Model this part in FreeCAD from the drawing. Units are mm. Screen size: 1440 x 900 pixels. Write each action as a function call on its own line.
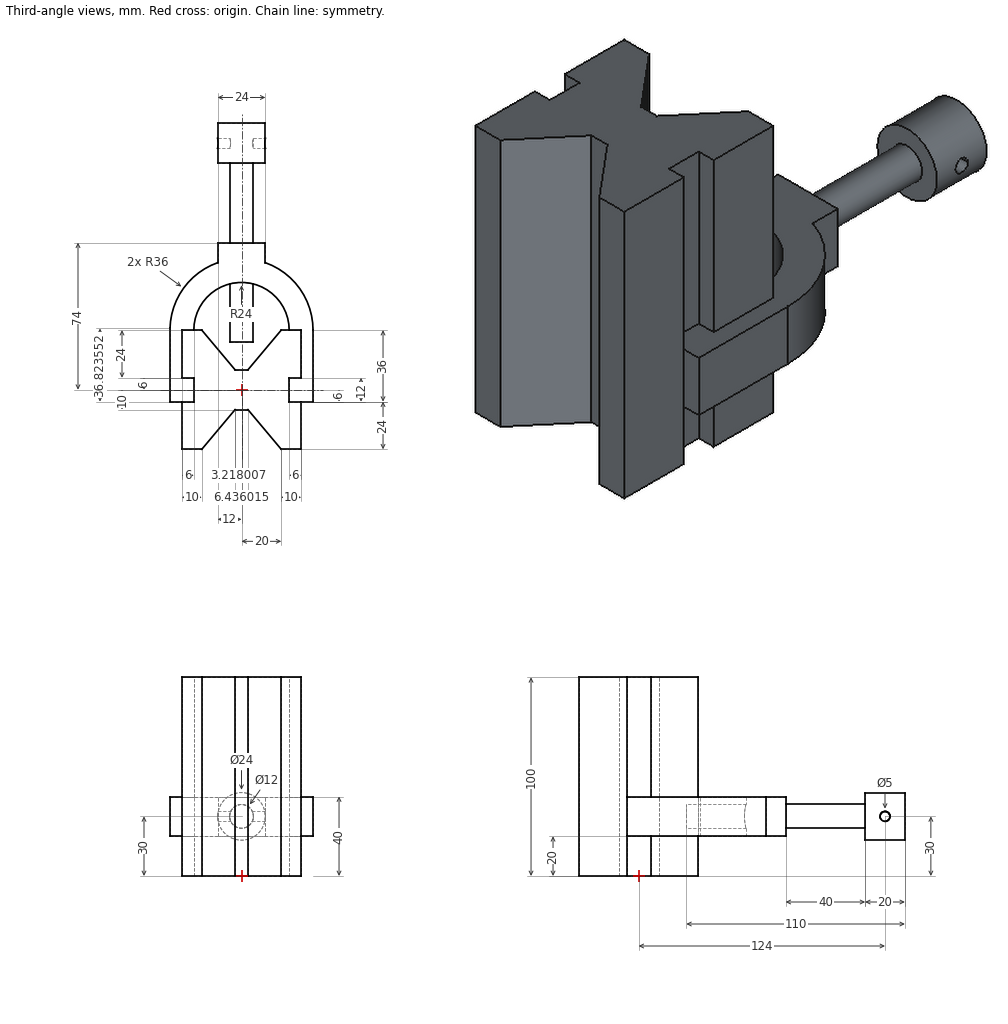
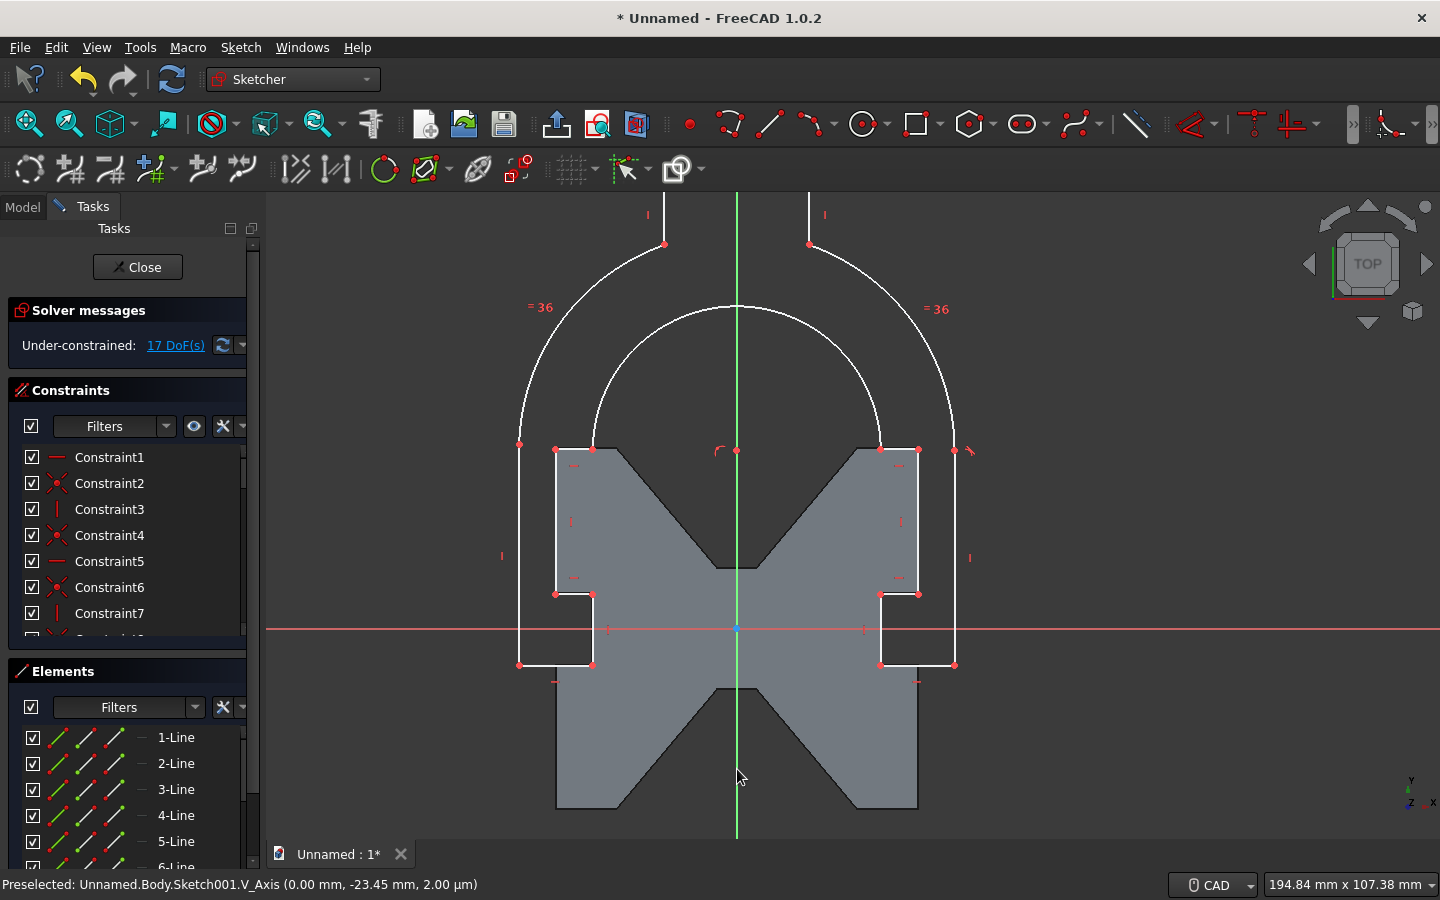
click(593, 666)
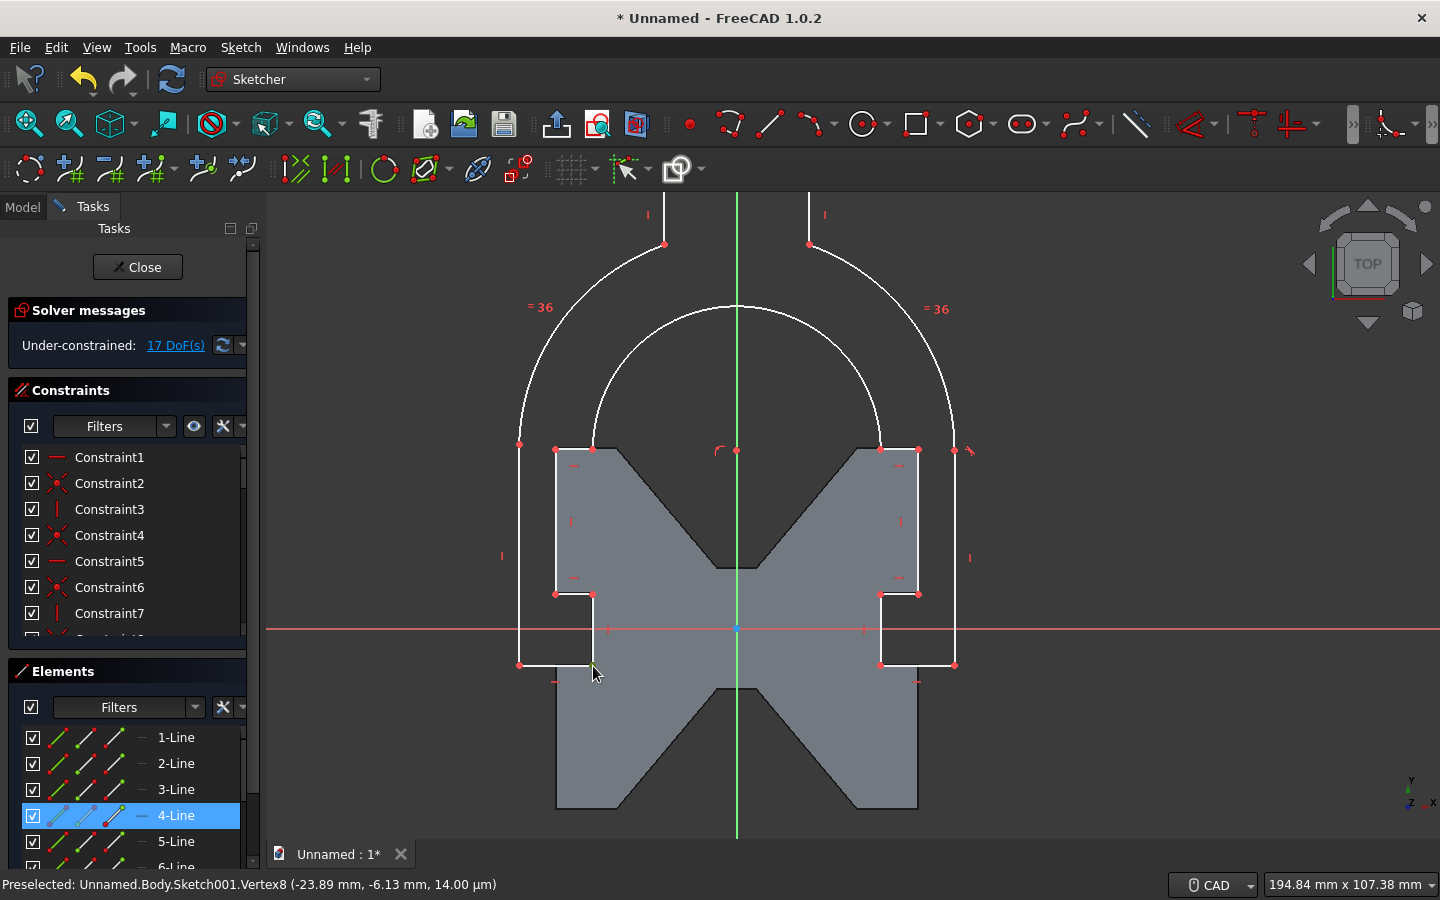
click(881, 666)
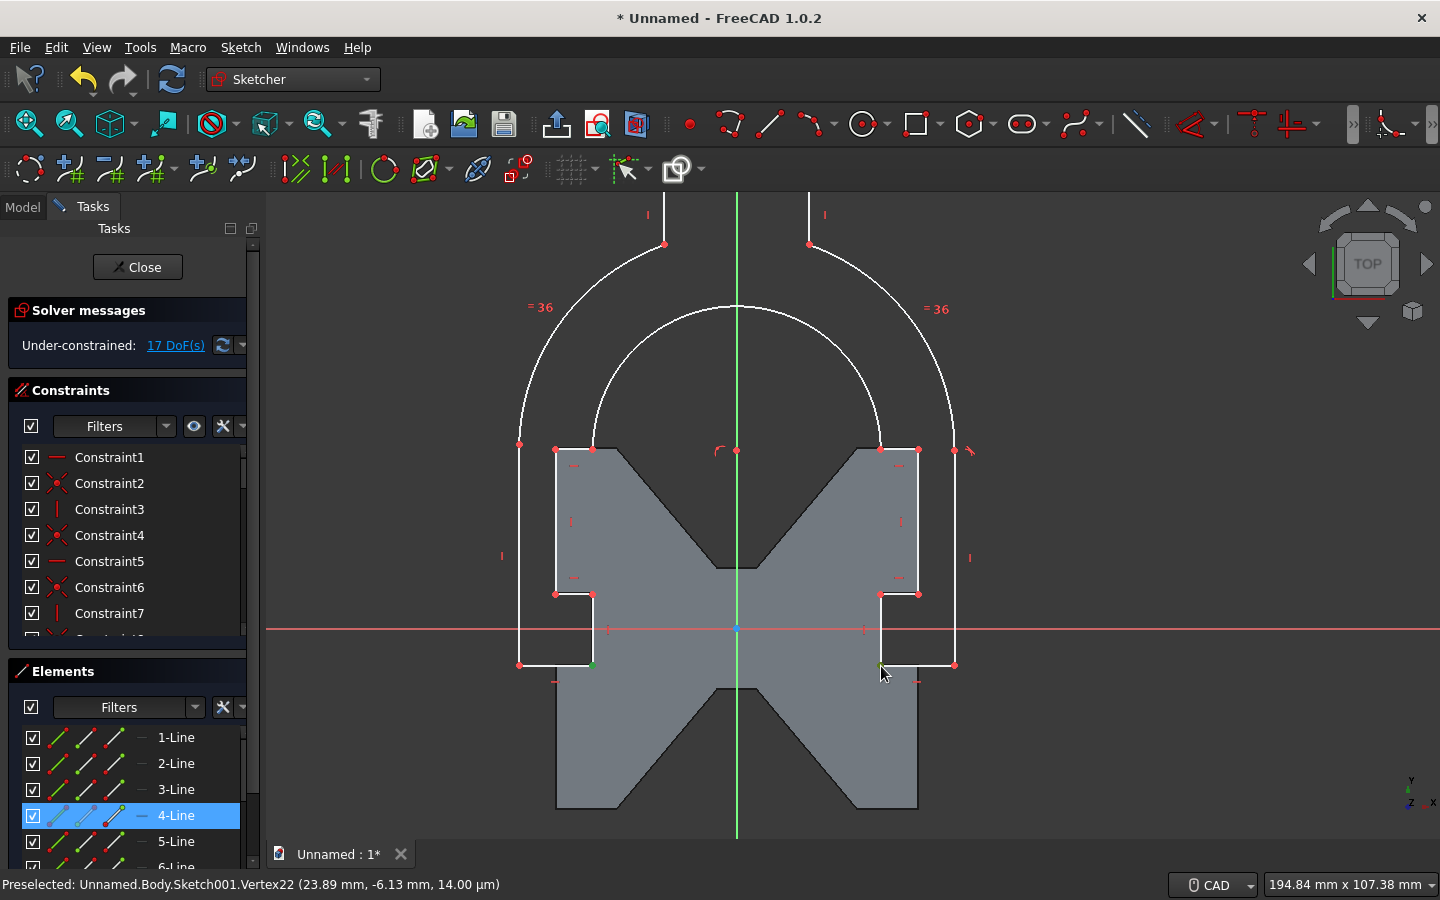
click(737, 769)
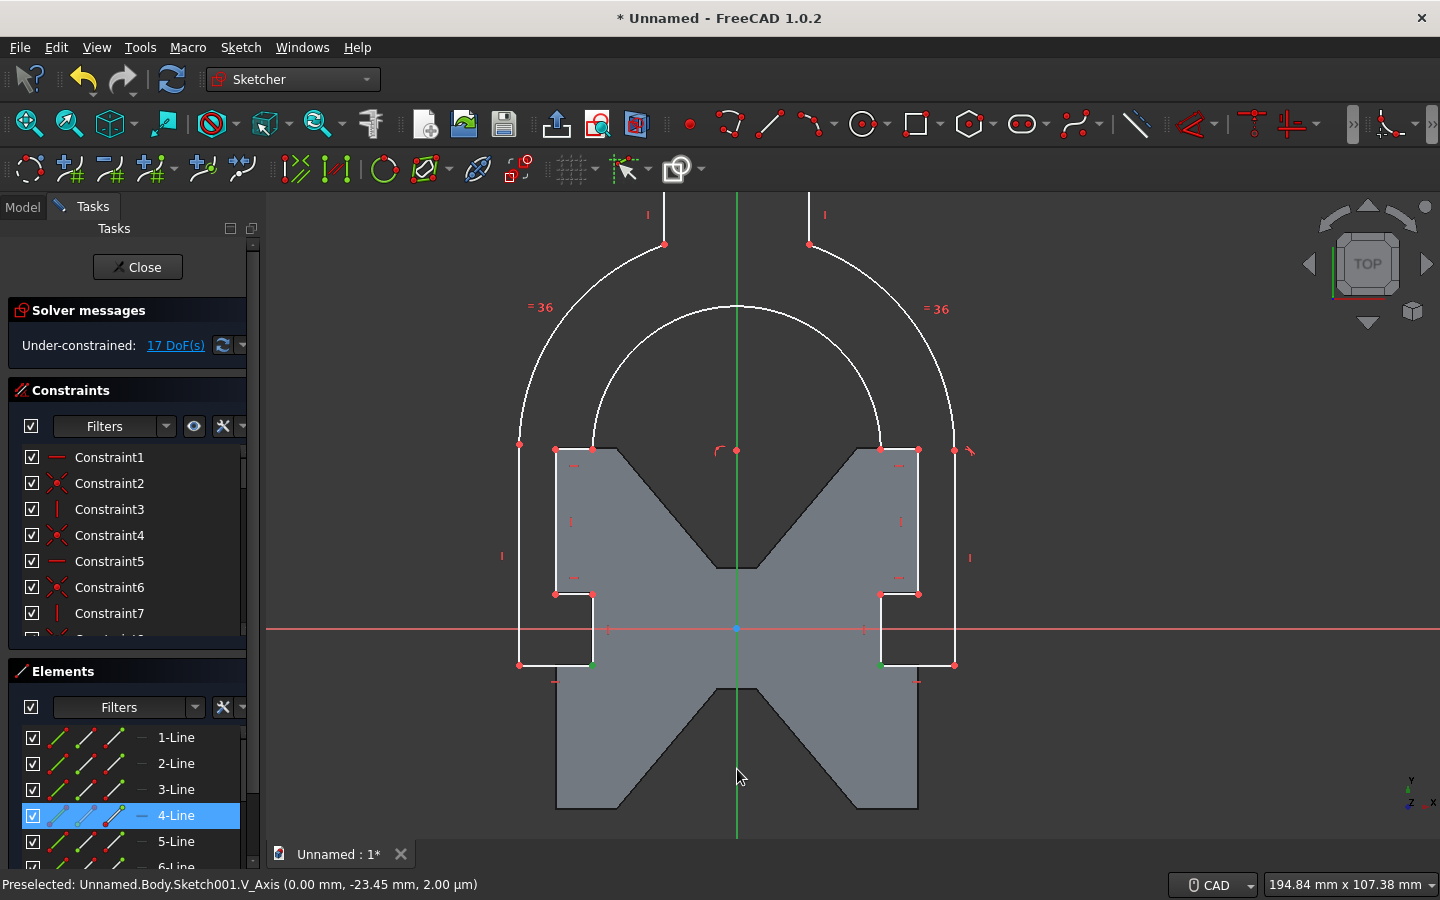
key(s)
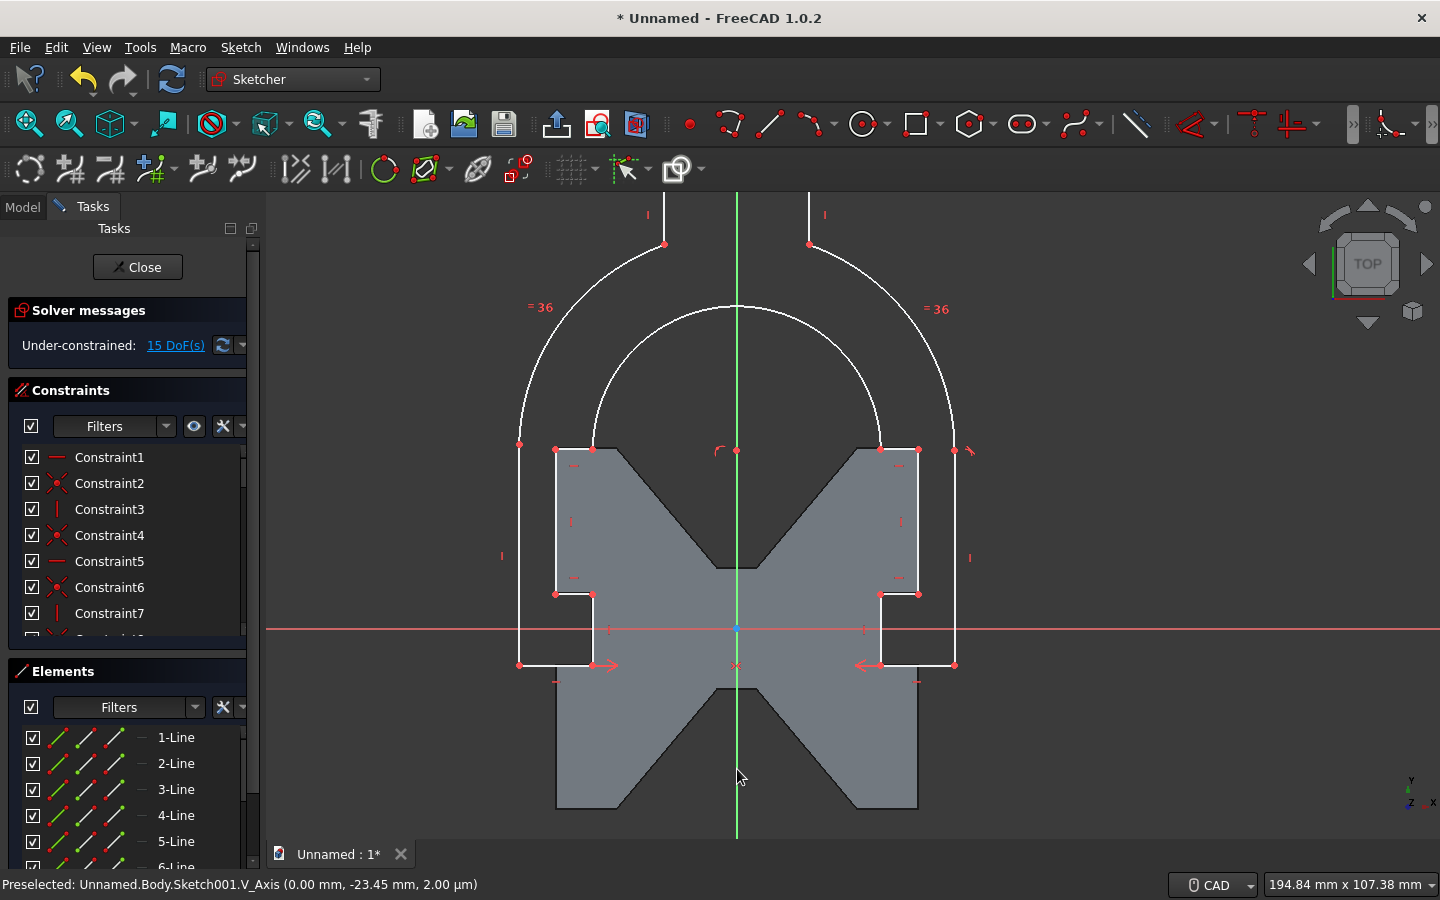
click(556, 594)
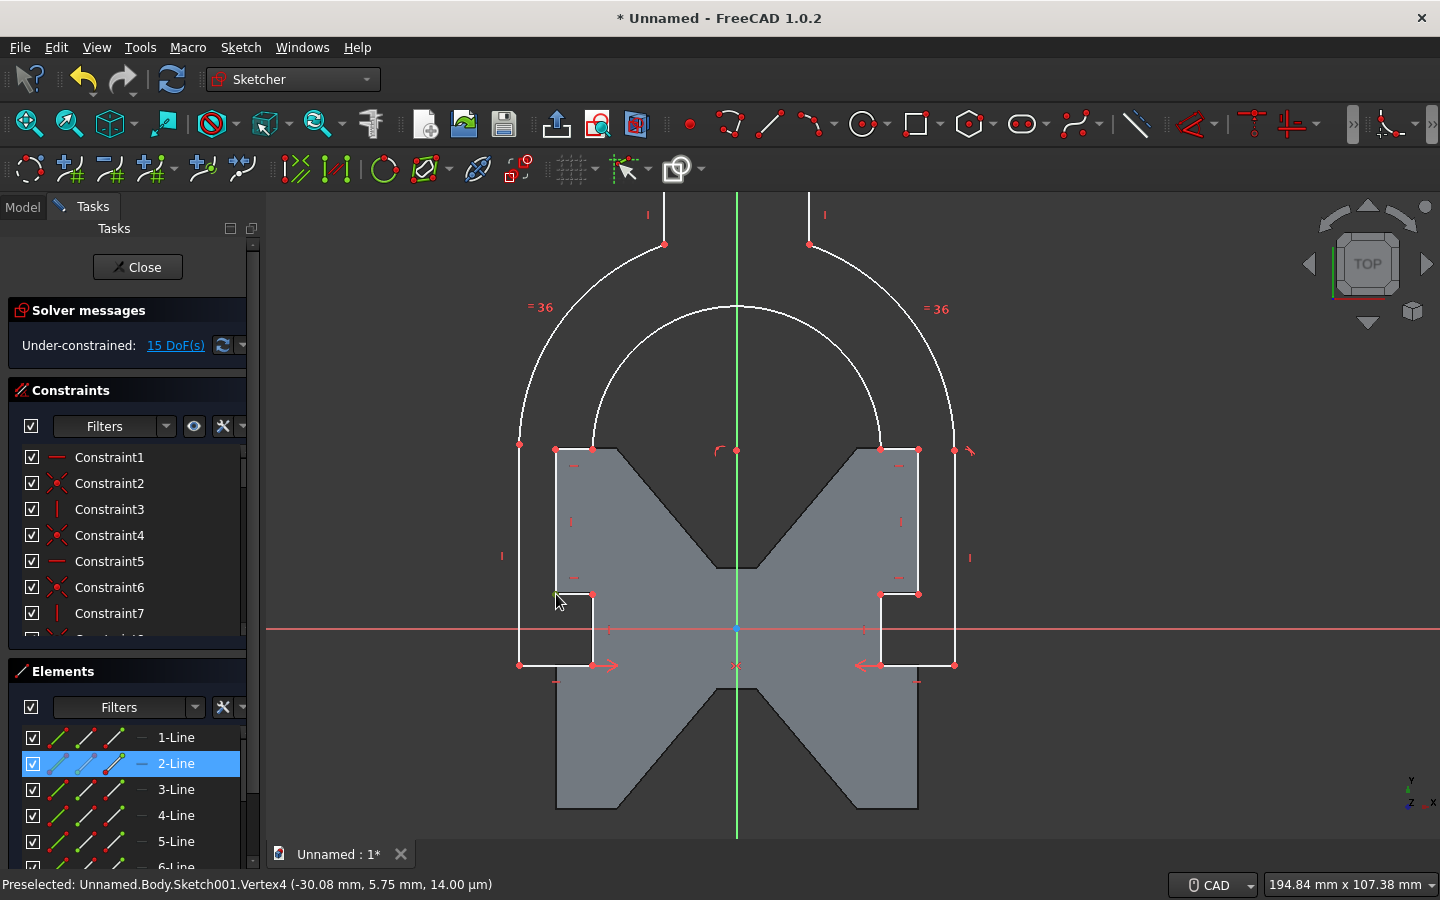
click(918, 594)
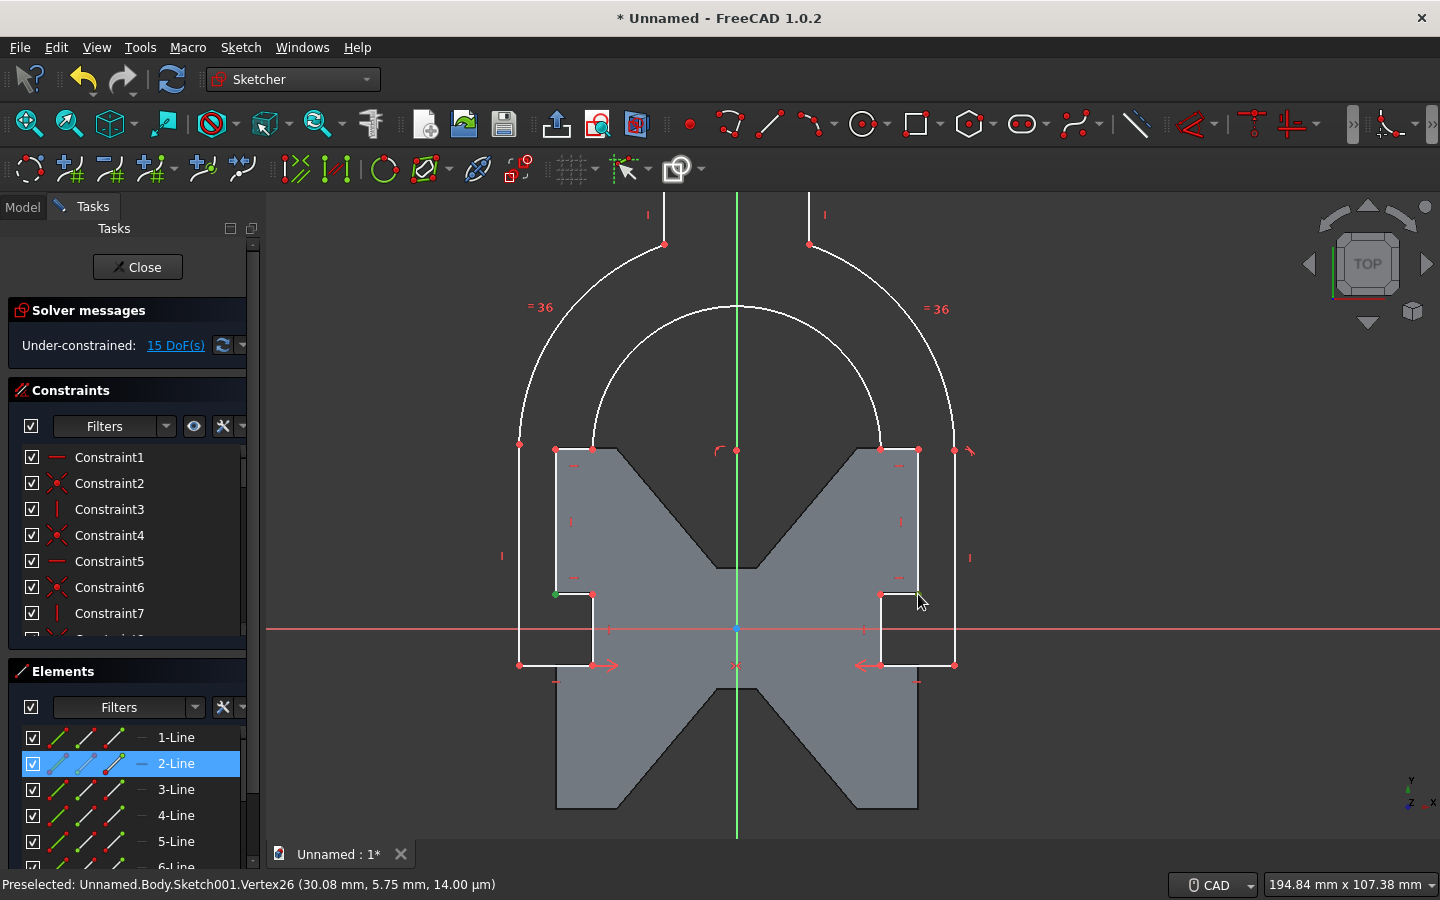
click(737, 769)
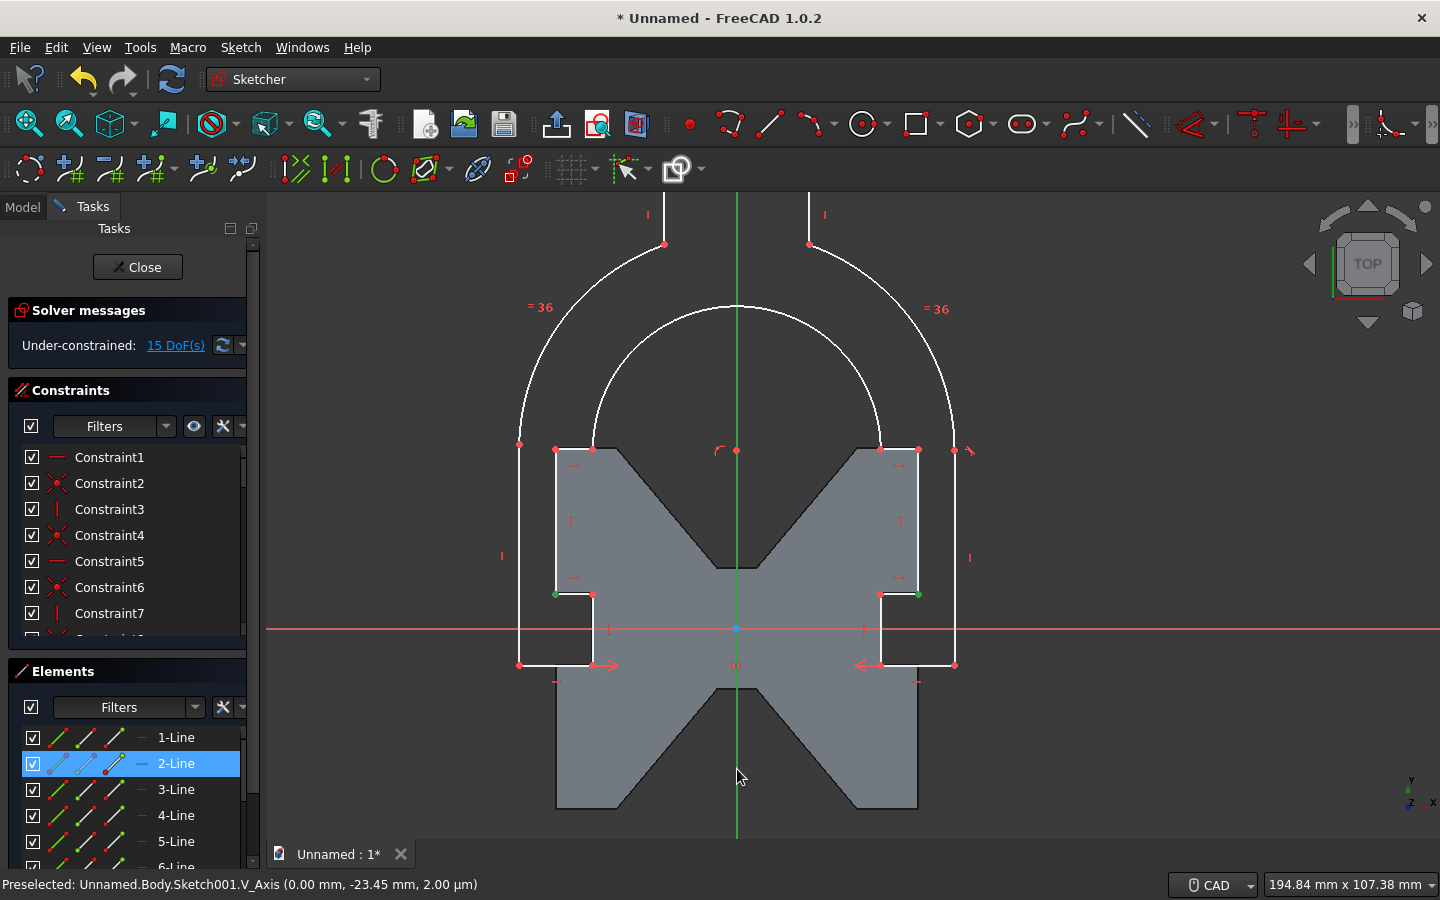
key(s)